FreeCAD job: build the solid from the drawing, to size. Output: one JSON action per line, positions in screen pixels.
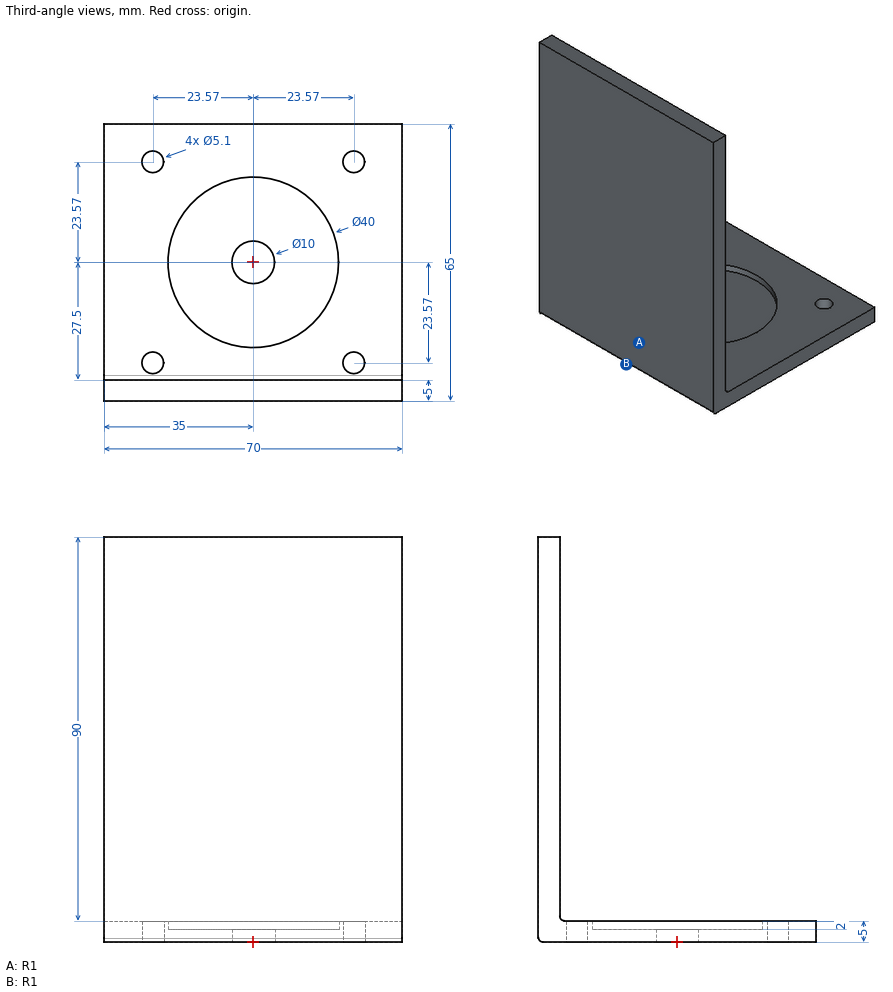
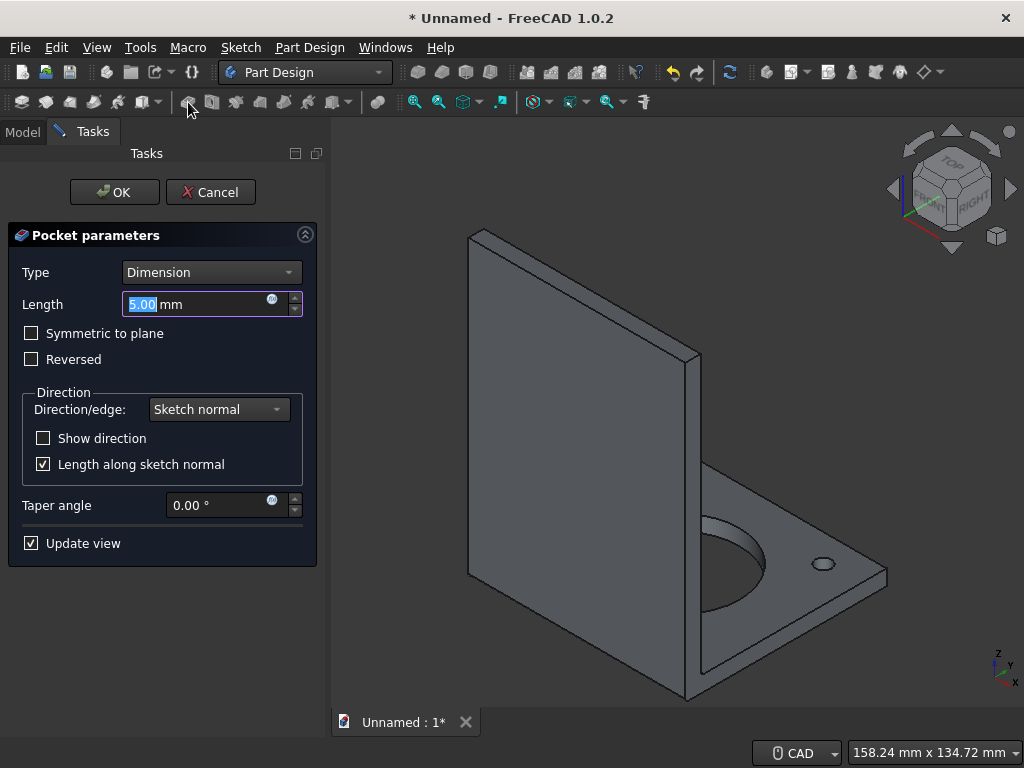
{"action": "type", "text": "2"}
{"action": "key", "text": "Tab"}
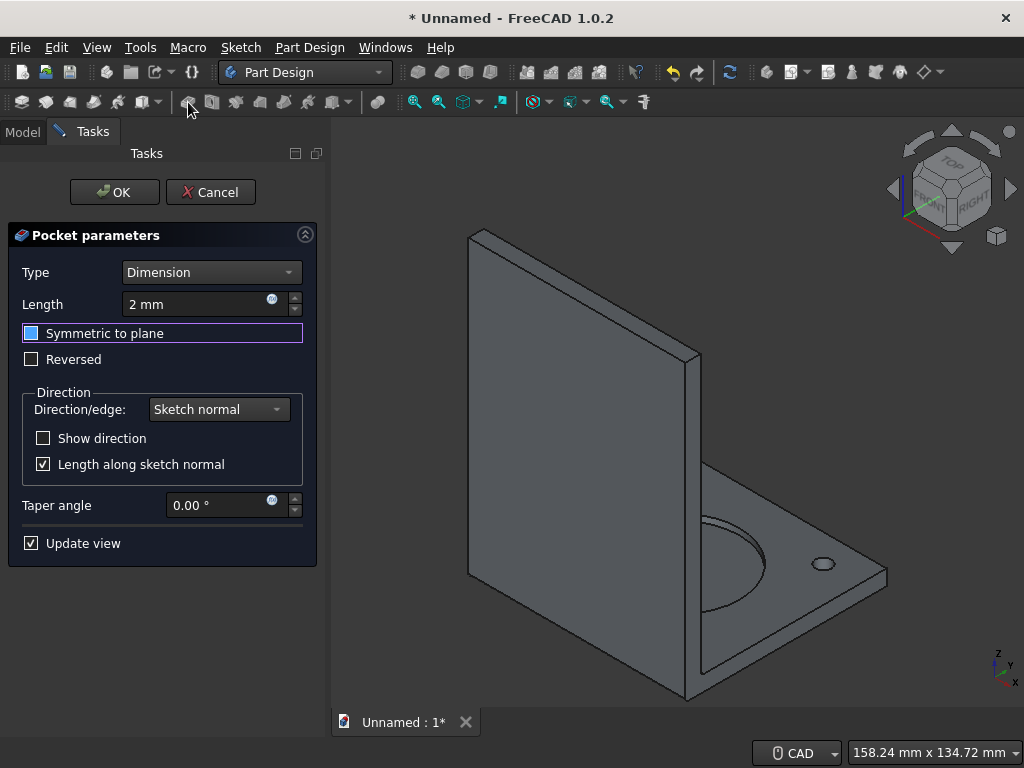
{"action": "left_click", "coordinate": [115, 192]}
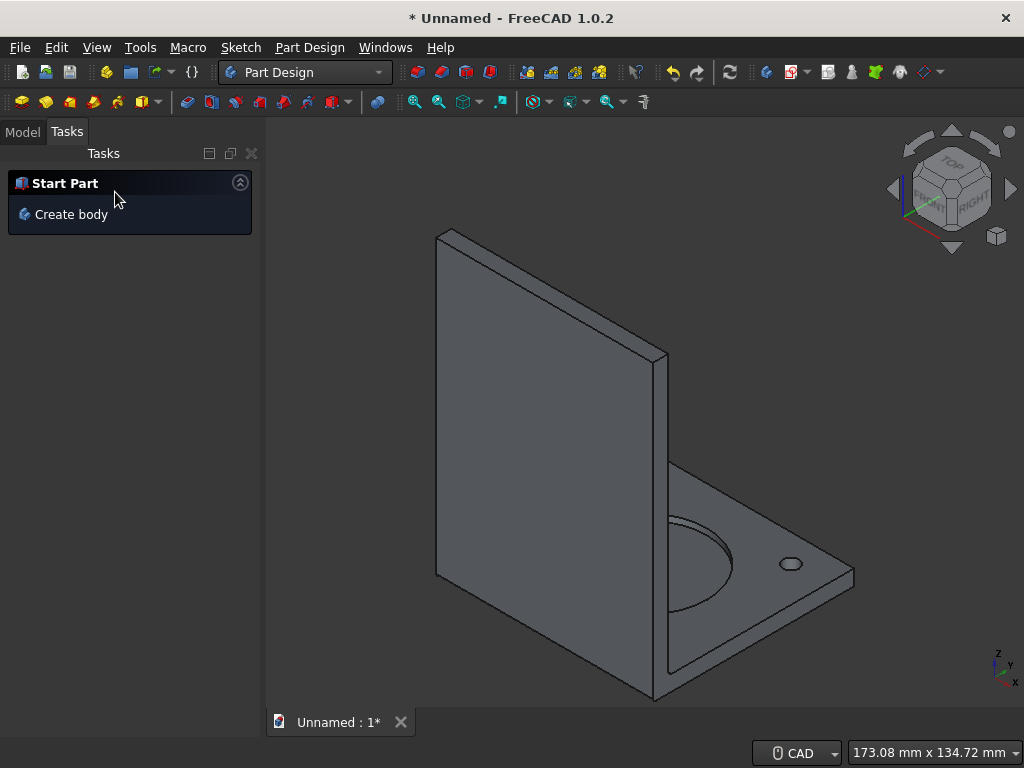
{"action": "left_click", "coordinate": [680, 570]}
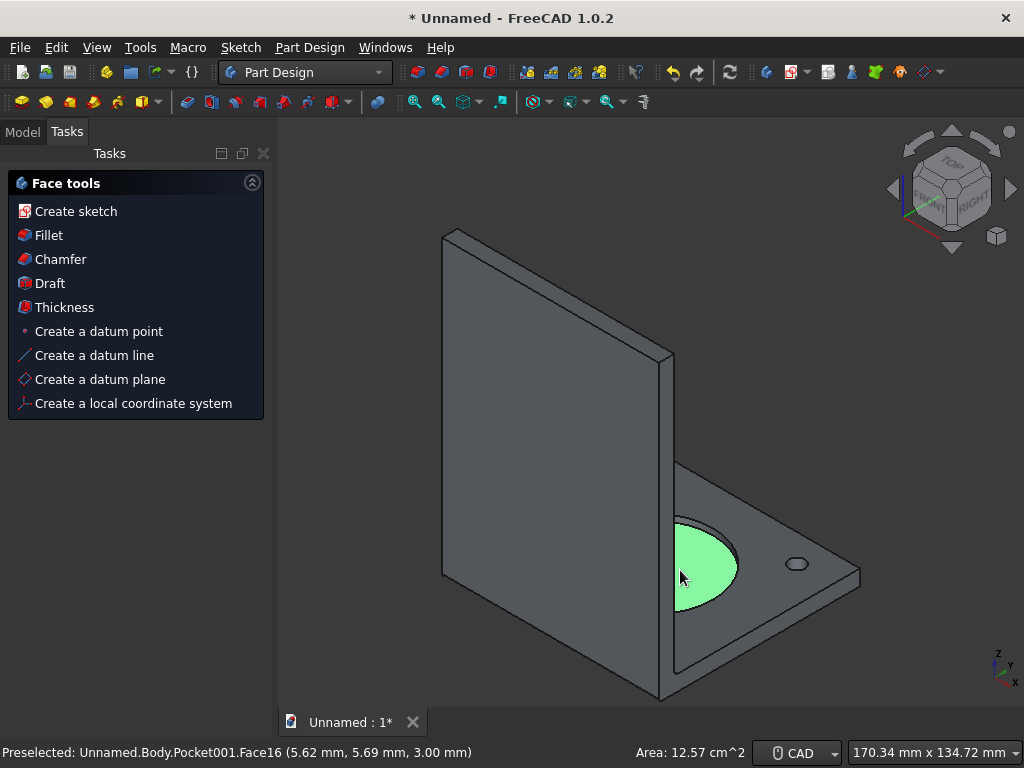
{"action": "left_click", "coordinate": [792, 72]}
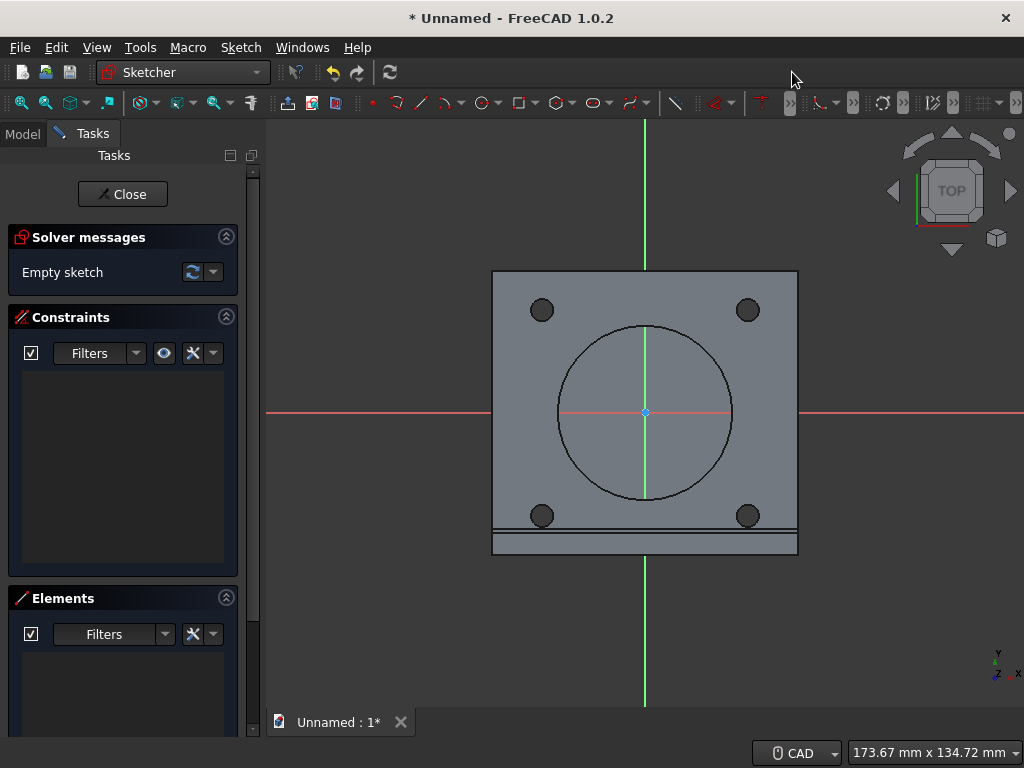
{"action": "left_click", "coordinate": [336, 104]}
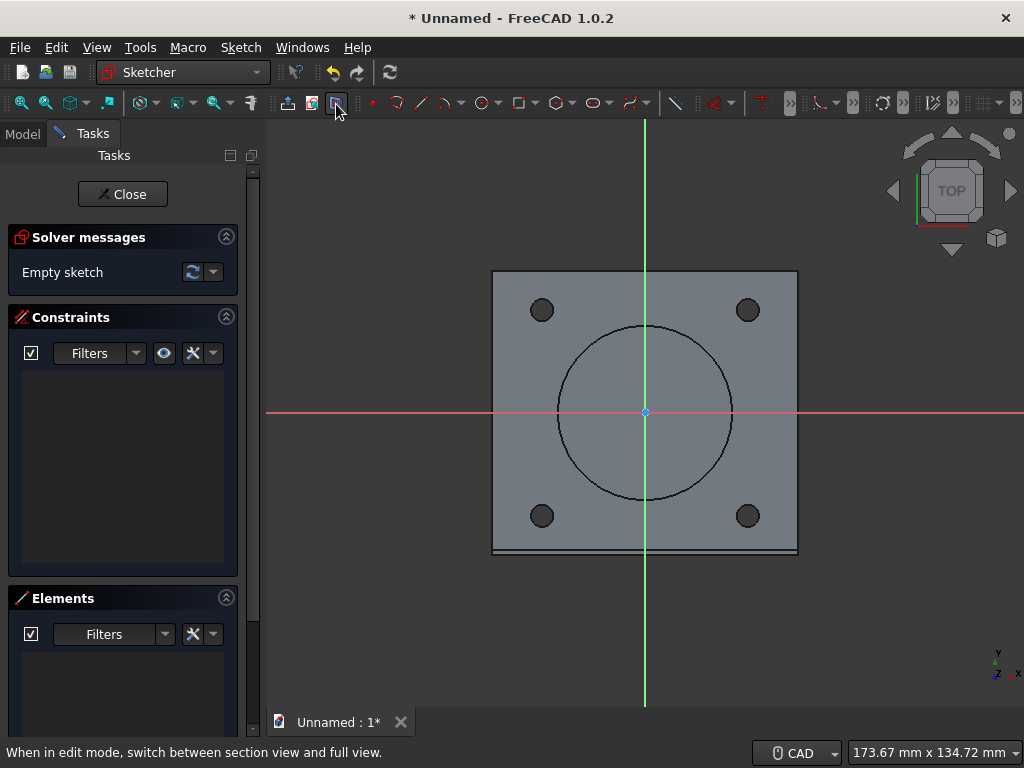
{"action": "scroll", "coordinate": [654, 413], "scroll_direction": "up", "scroll_amount": 11}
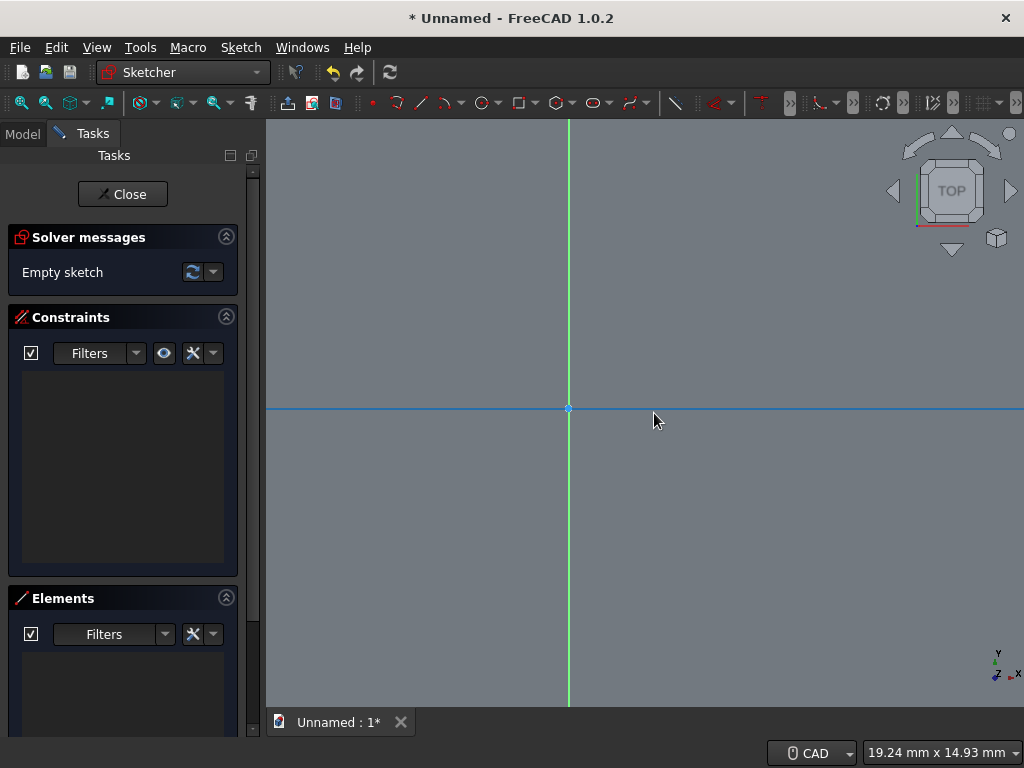
{"action": "left_click", "coordinate": [482, 104]}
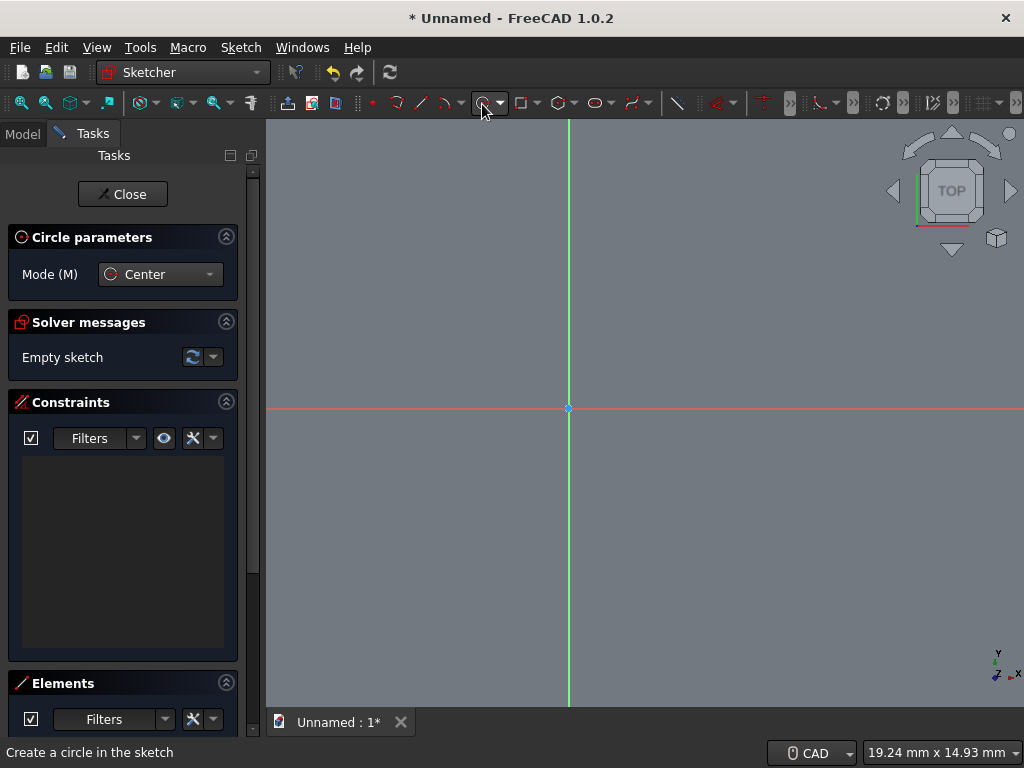
{"action": "left_click", "coordinate": [569, 409]}
{"action": "mouse_move", "coordinate": [708, 270]}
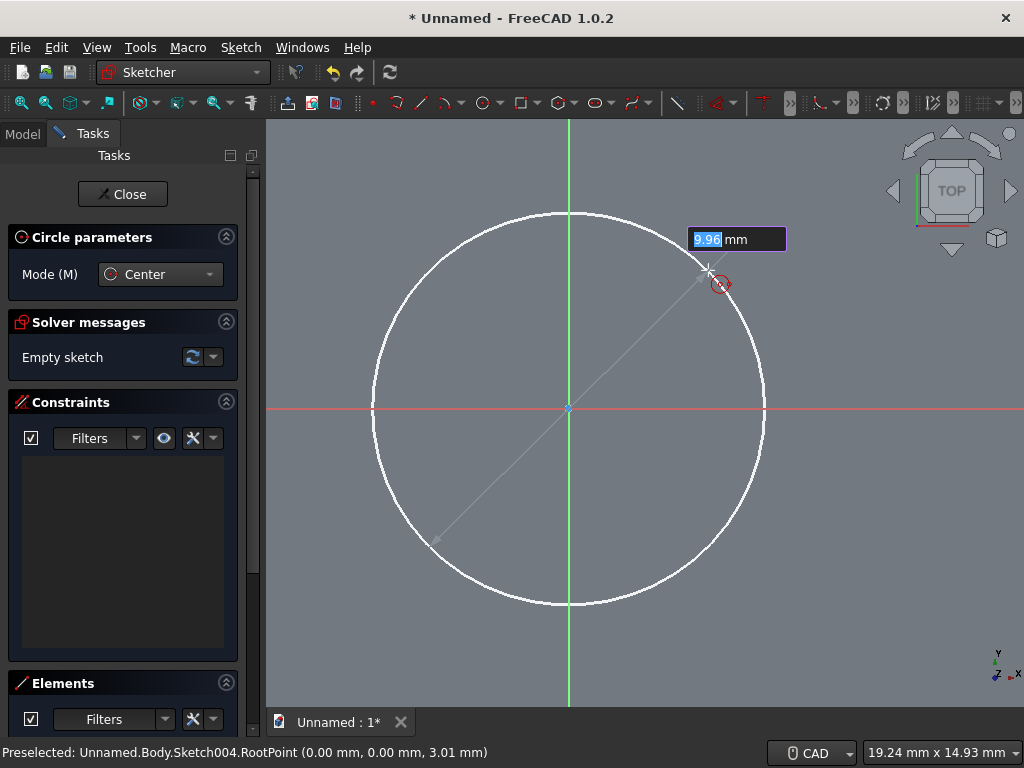
{"action": "type", "text": "10"}
{"action": "key", "text": "Return"}
{"action": "key", "text": "Escape"}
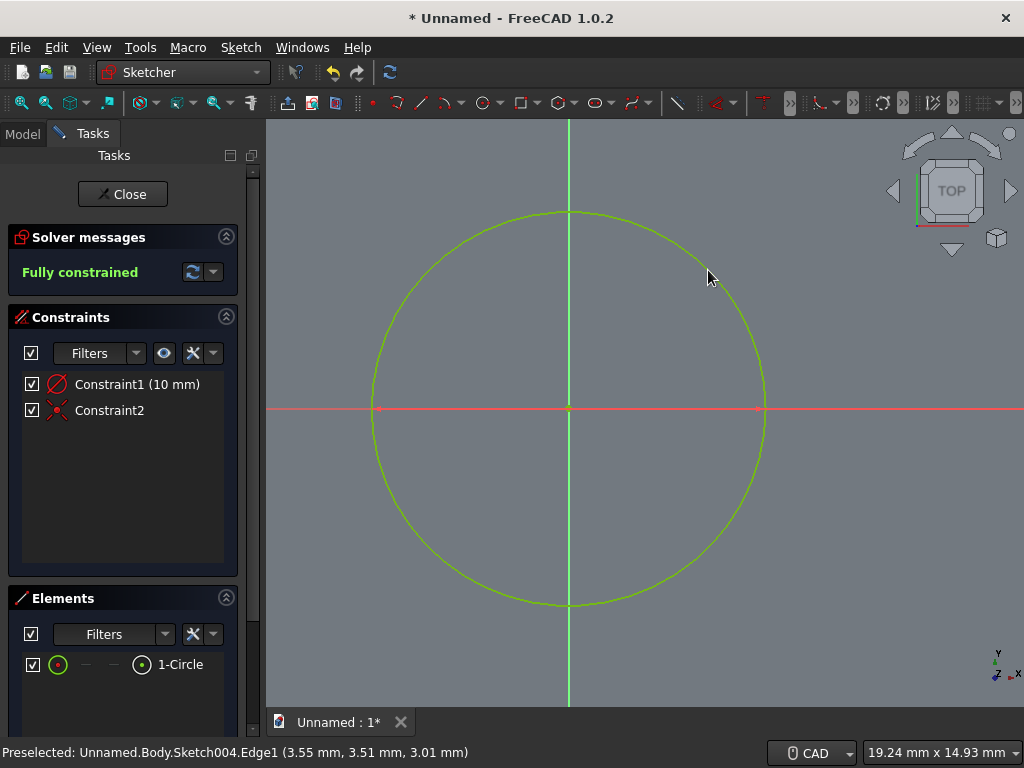
{"action": "left_click", "coordinate": [123, 194]}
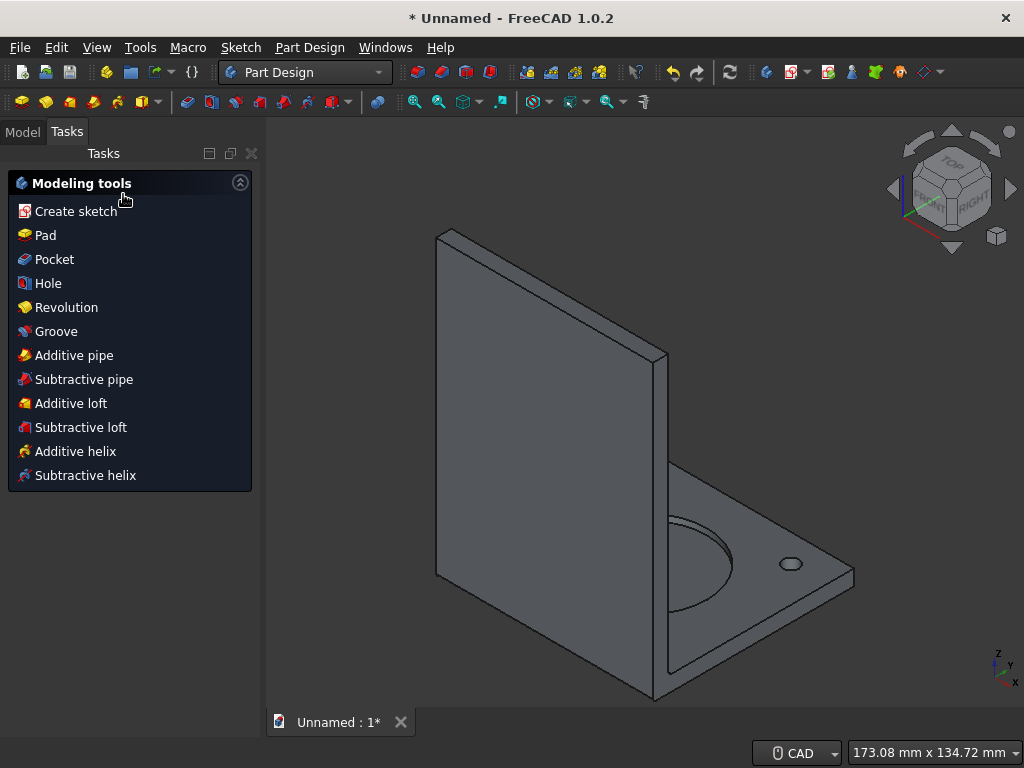
{"action": "left_click", "coordinate": [188, 102]}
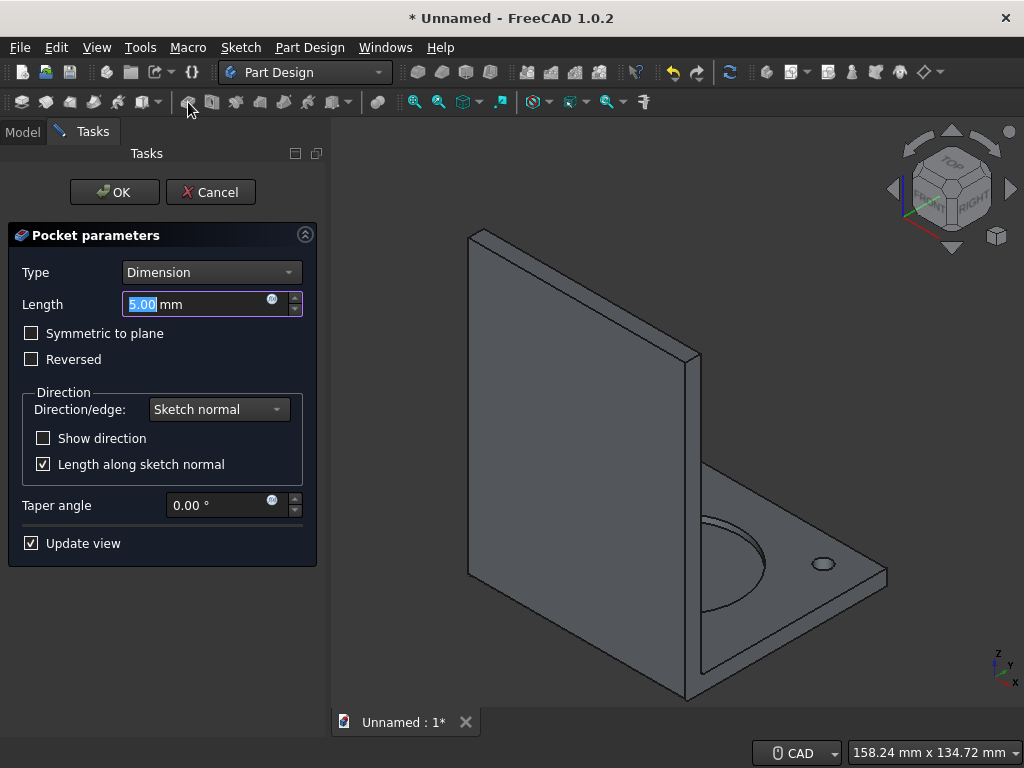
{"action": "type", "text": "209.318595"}
{"action": "key", "text": "Tab"}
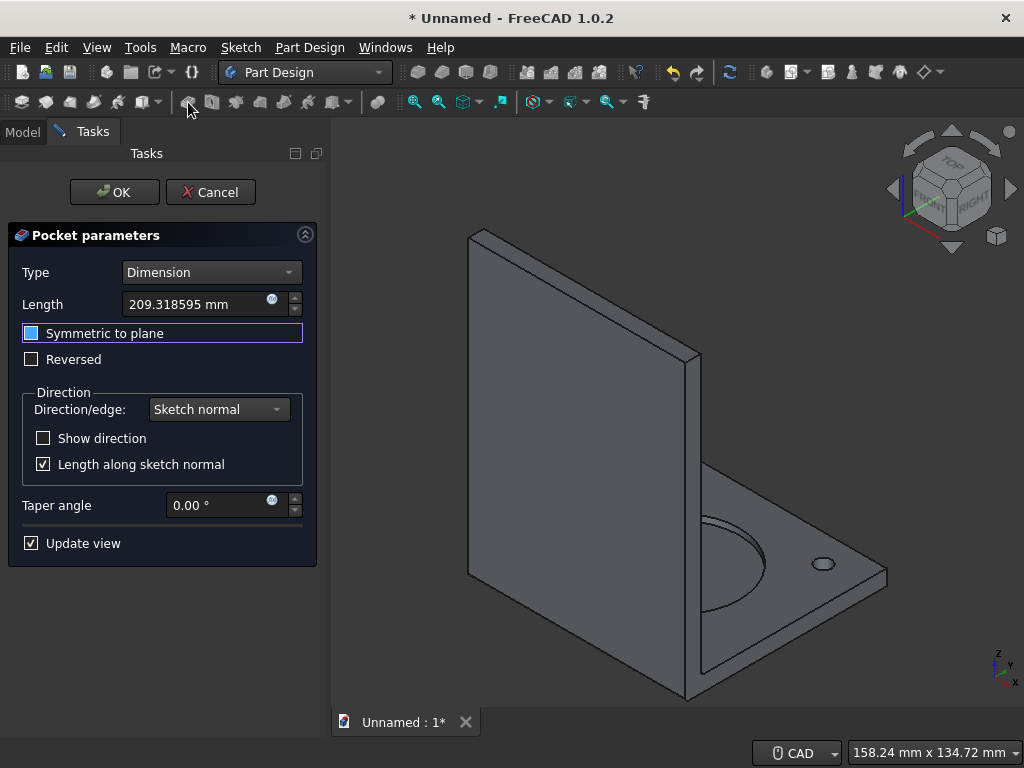
{"action": "left_click", "coordinate": [30, 333]}